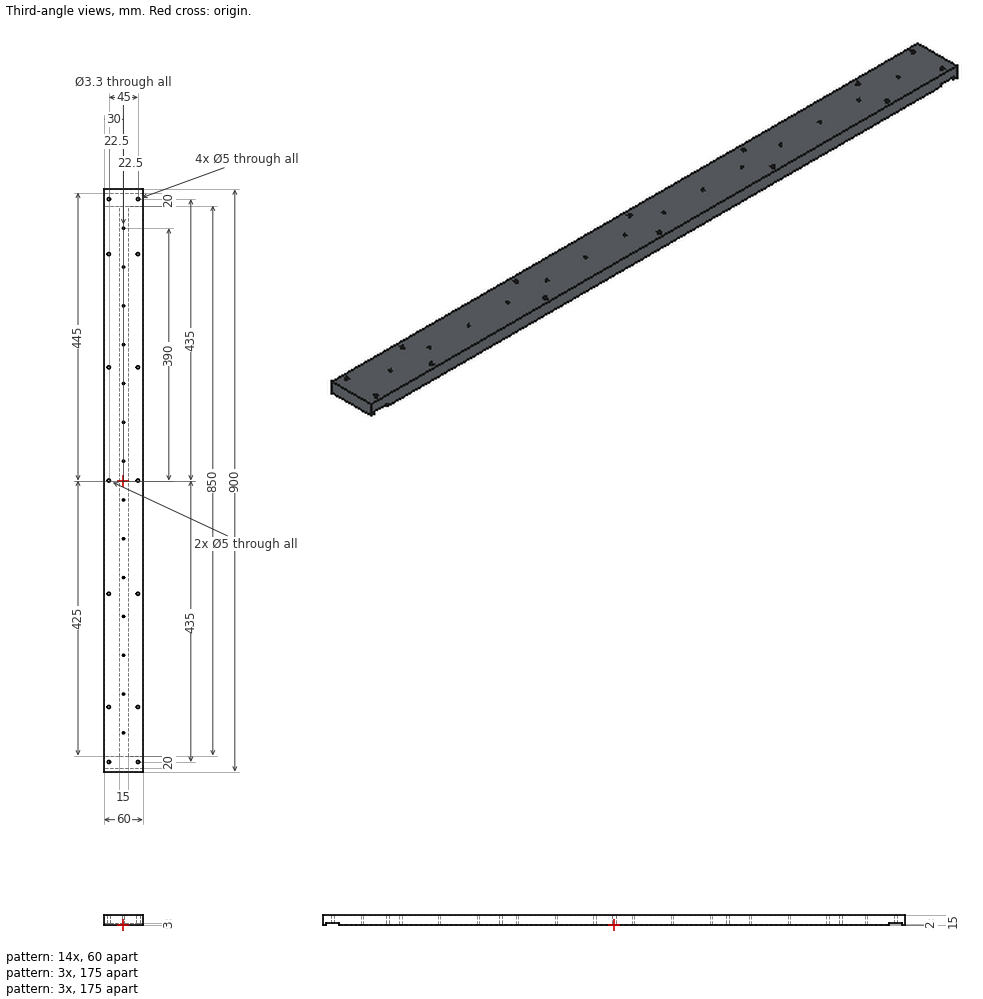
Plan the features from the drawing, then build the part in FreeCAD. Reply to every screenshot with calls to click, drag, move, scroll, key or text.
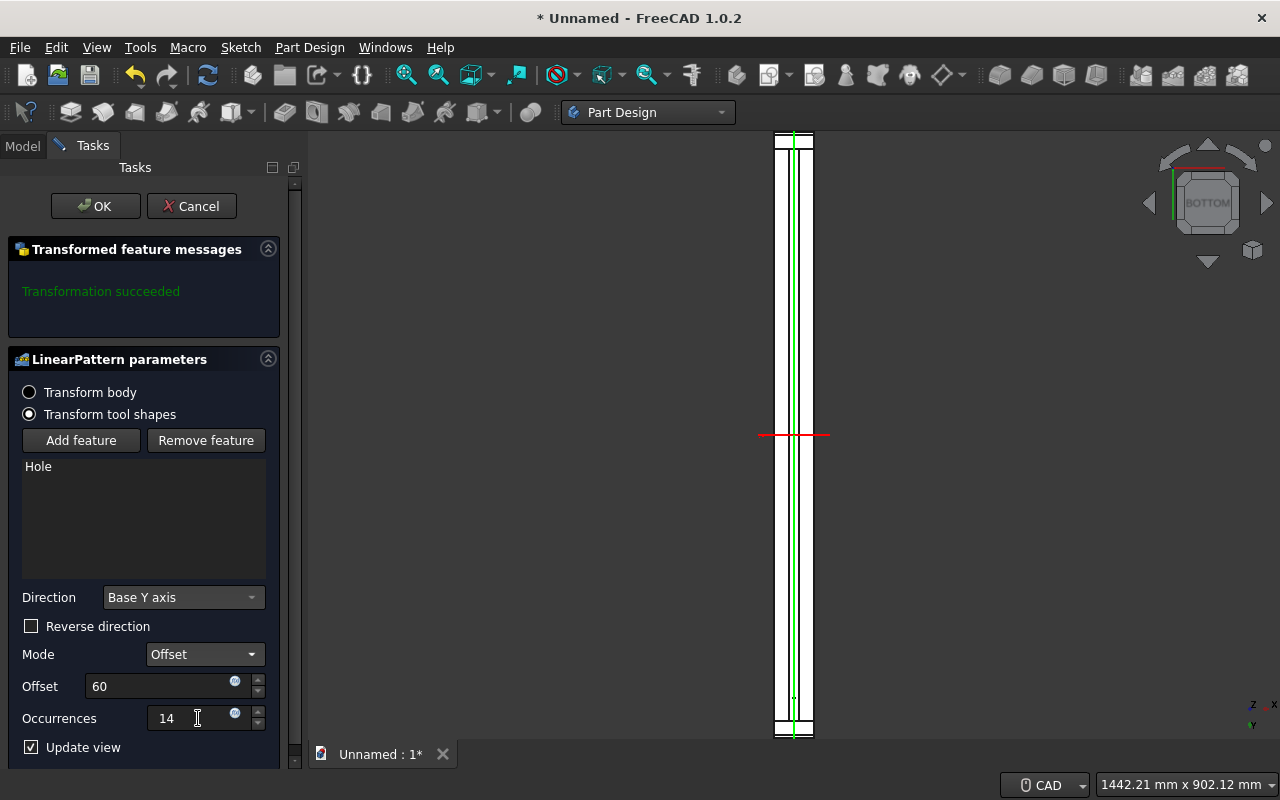
click(30, 626)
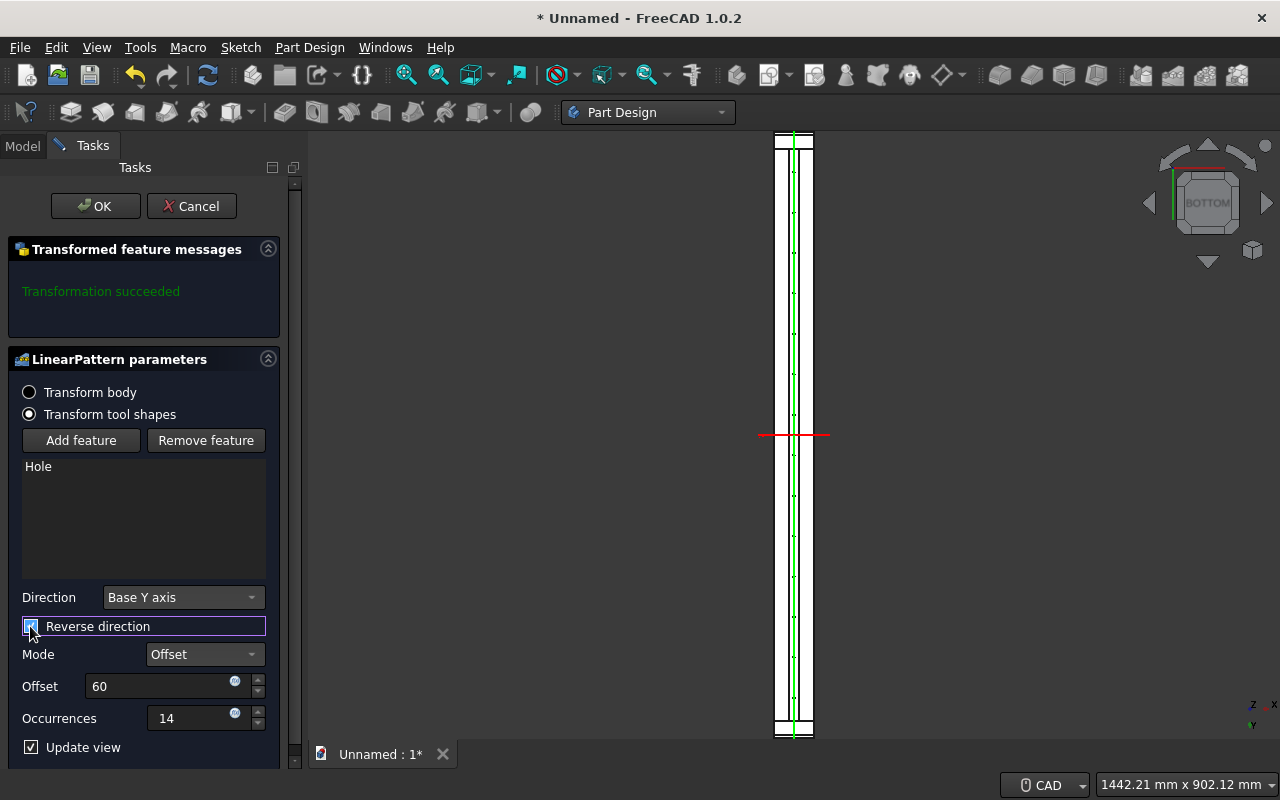
click(96, 206)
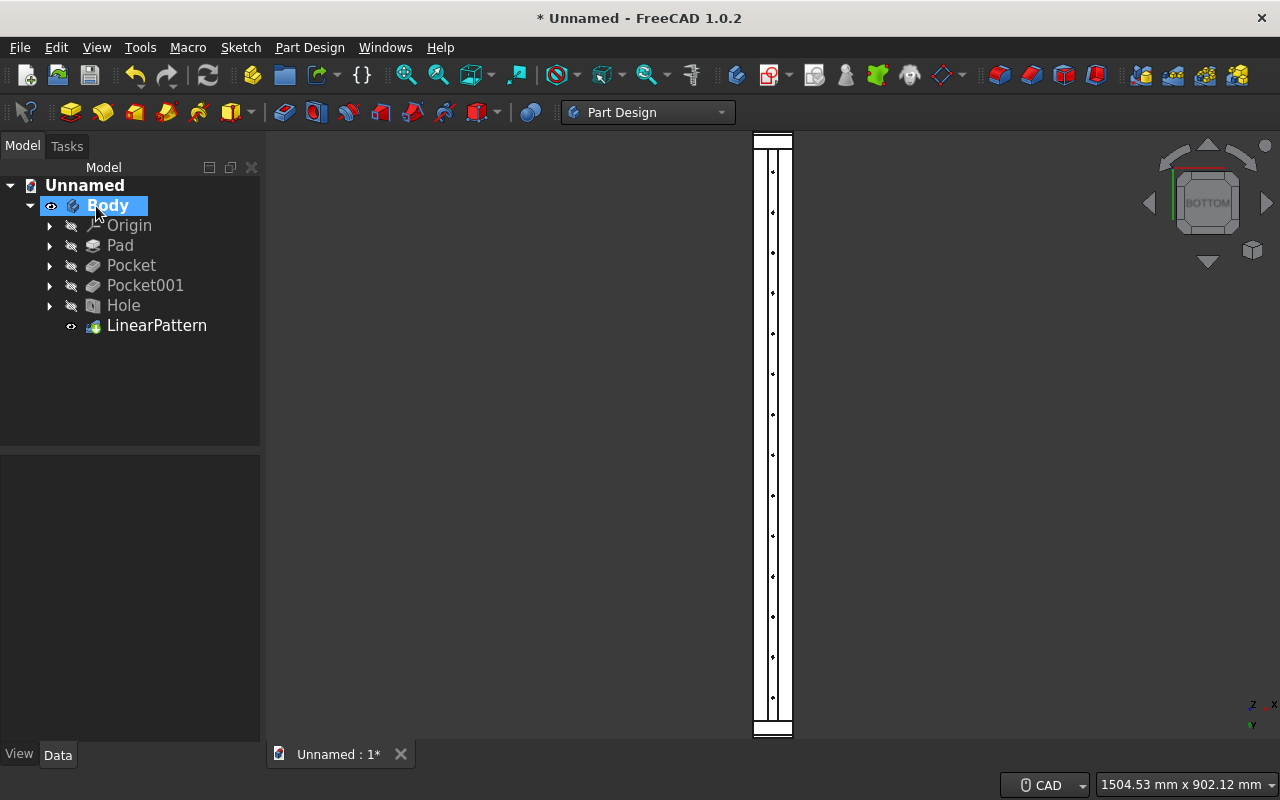
key(1)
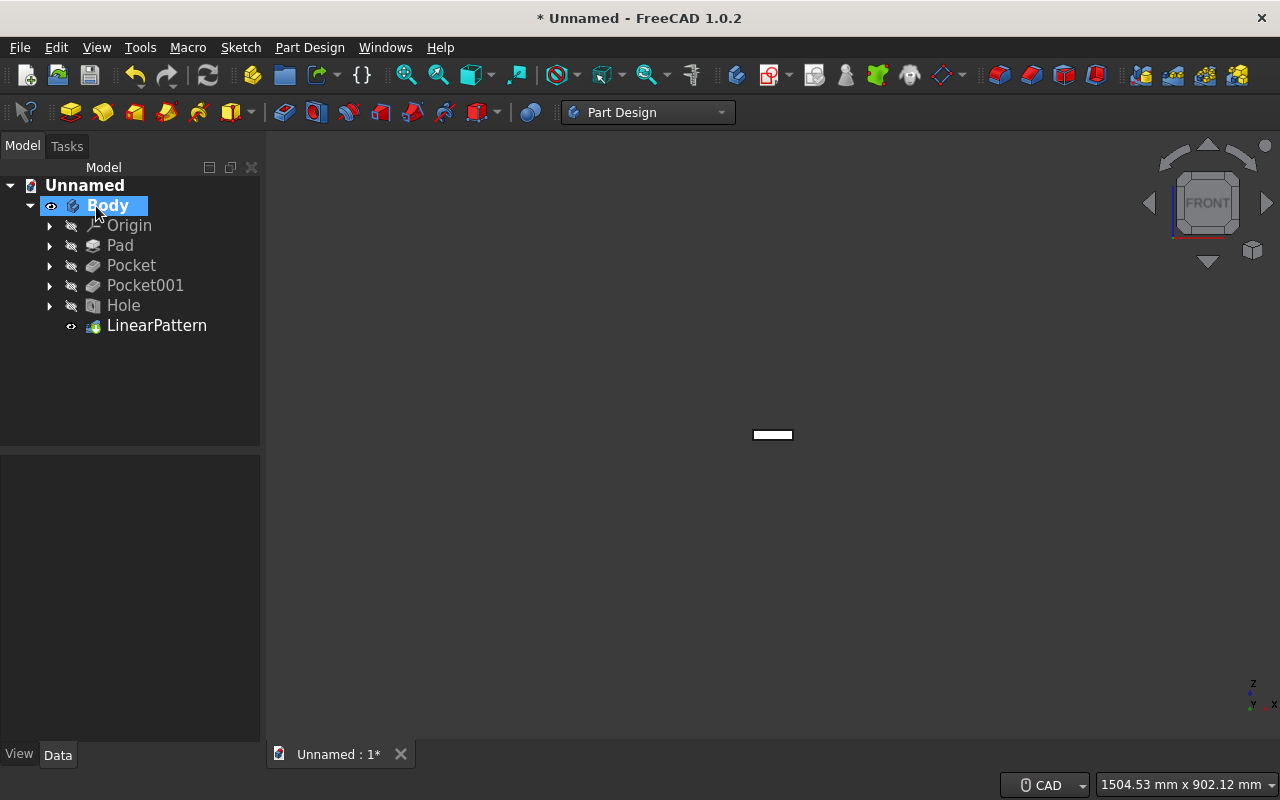
key(v)
key(f)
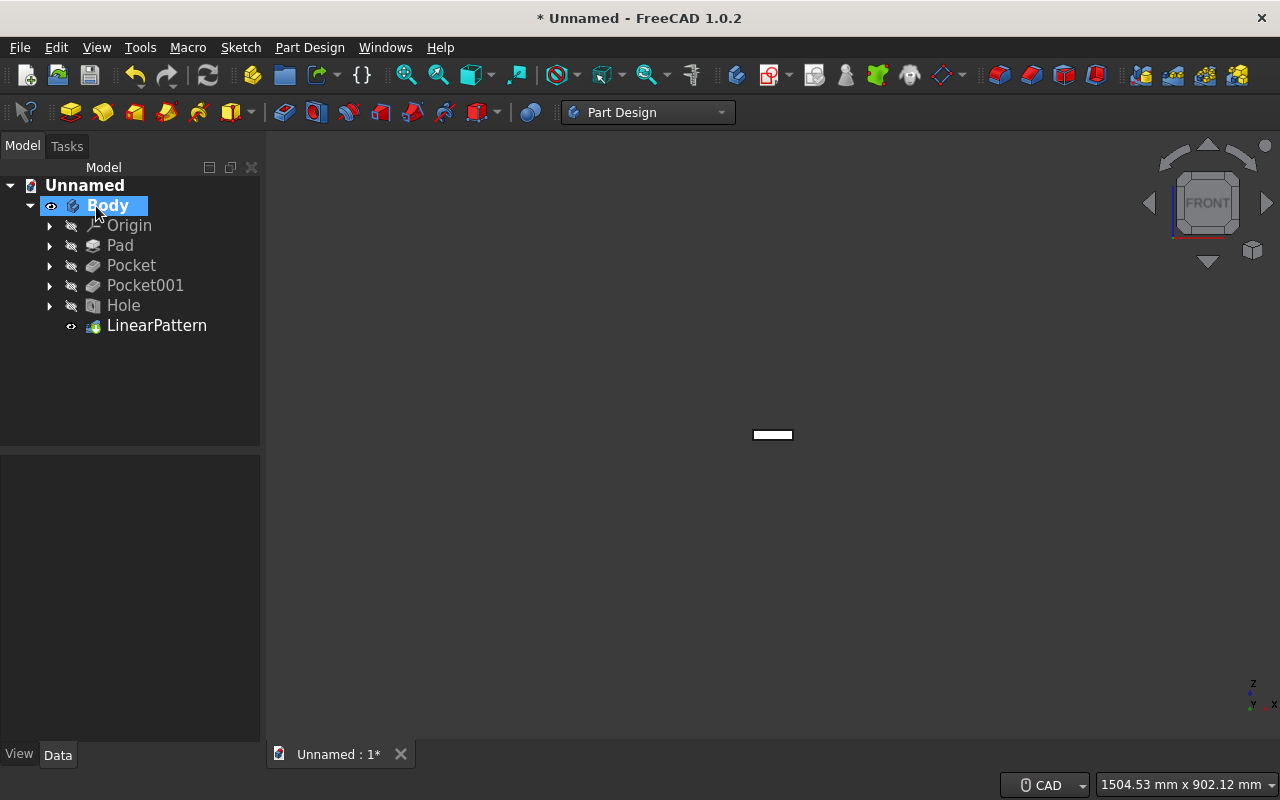
key(5)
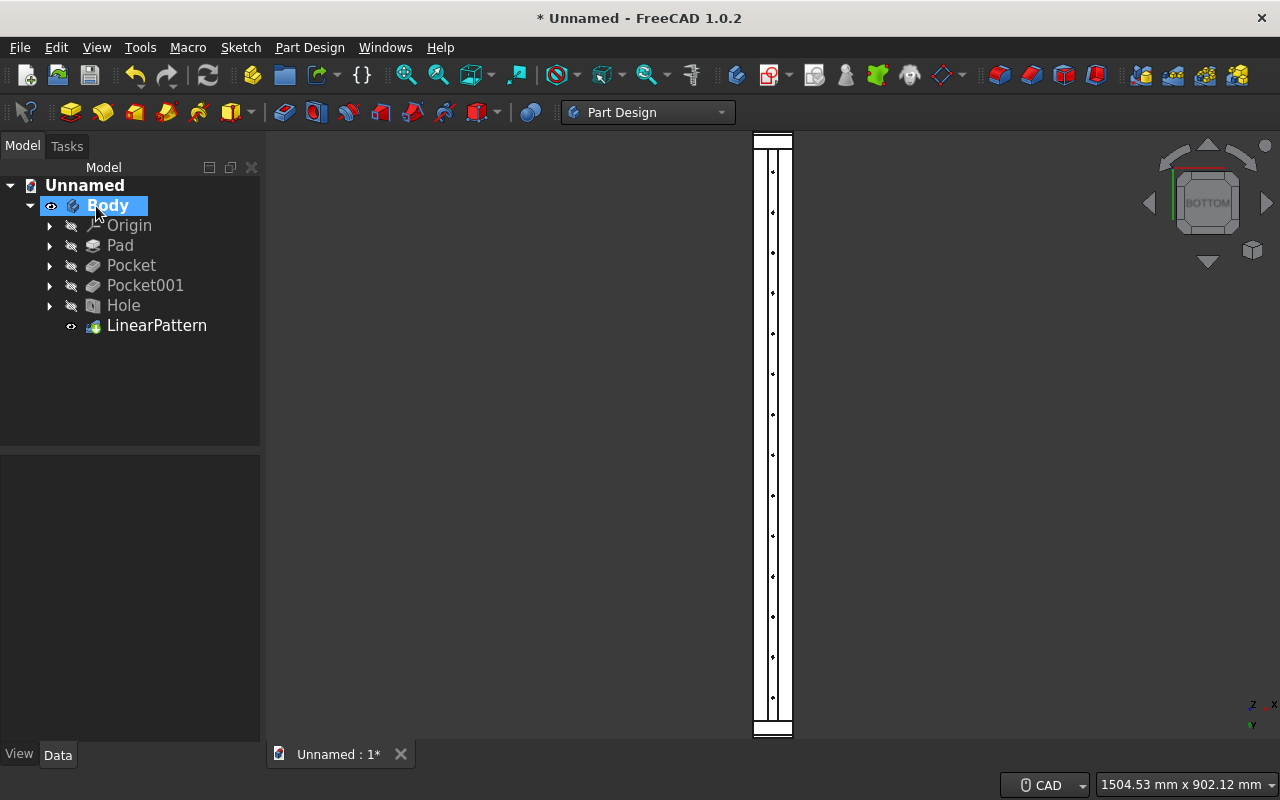
key(3)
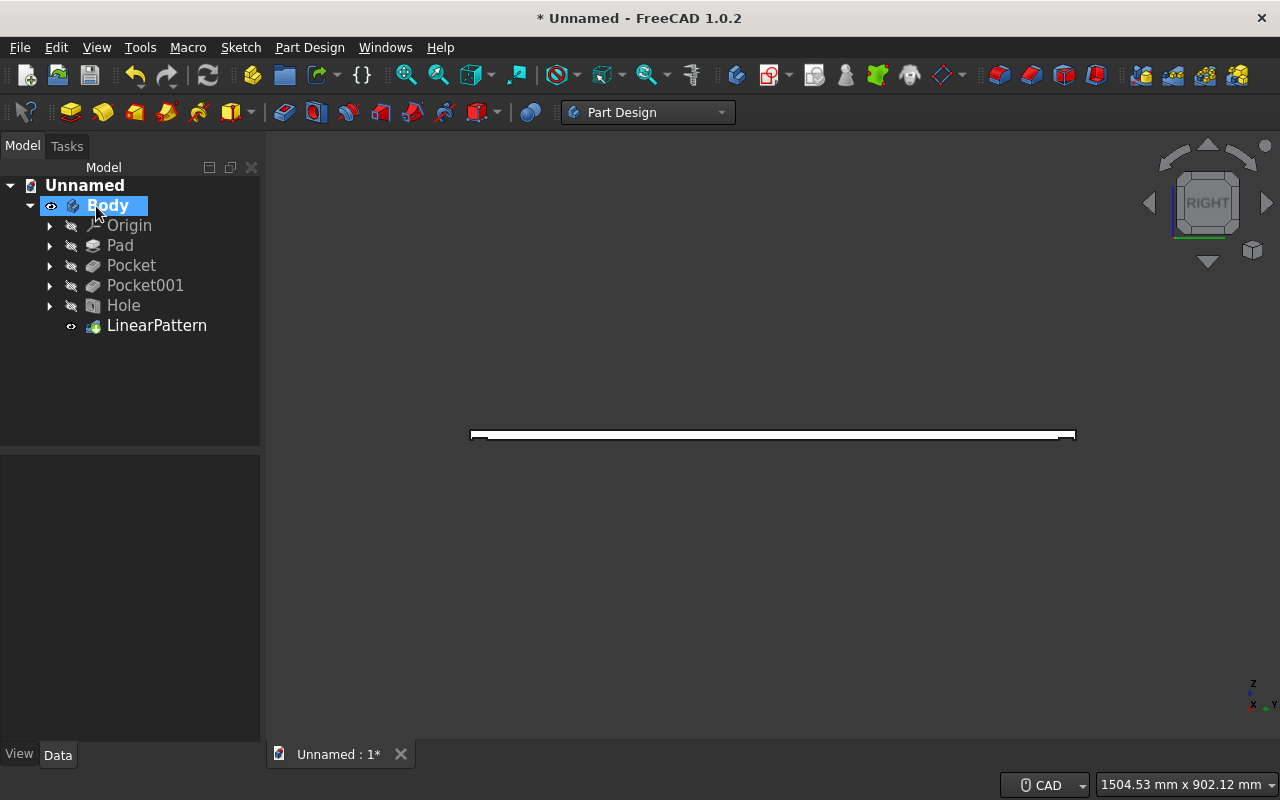
click(50, 226)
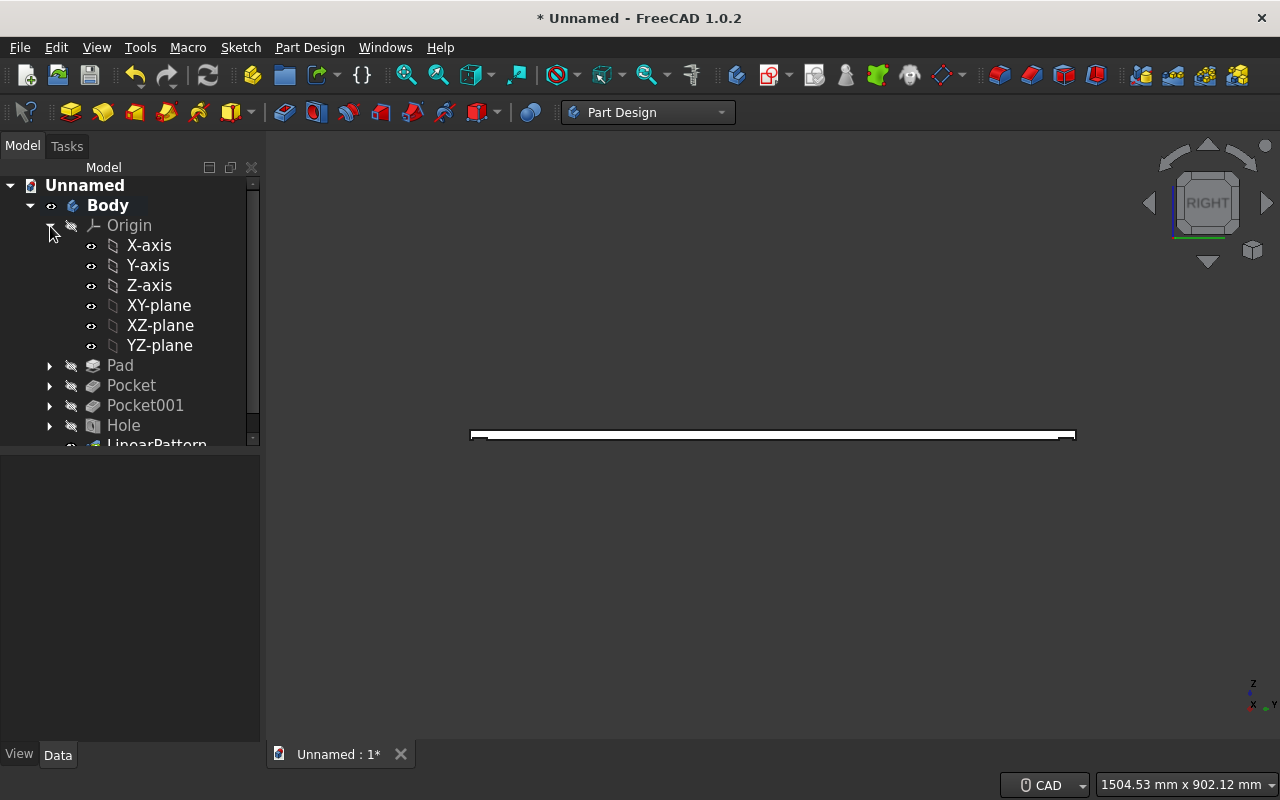
click(136, 306)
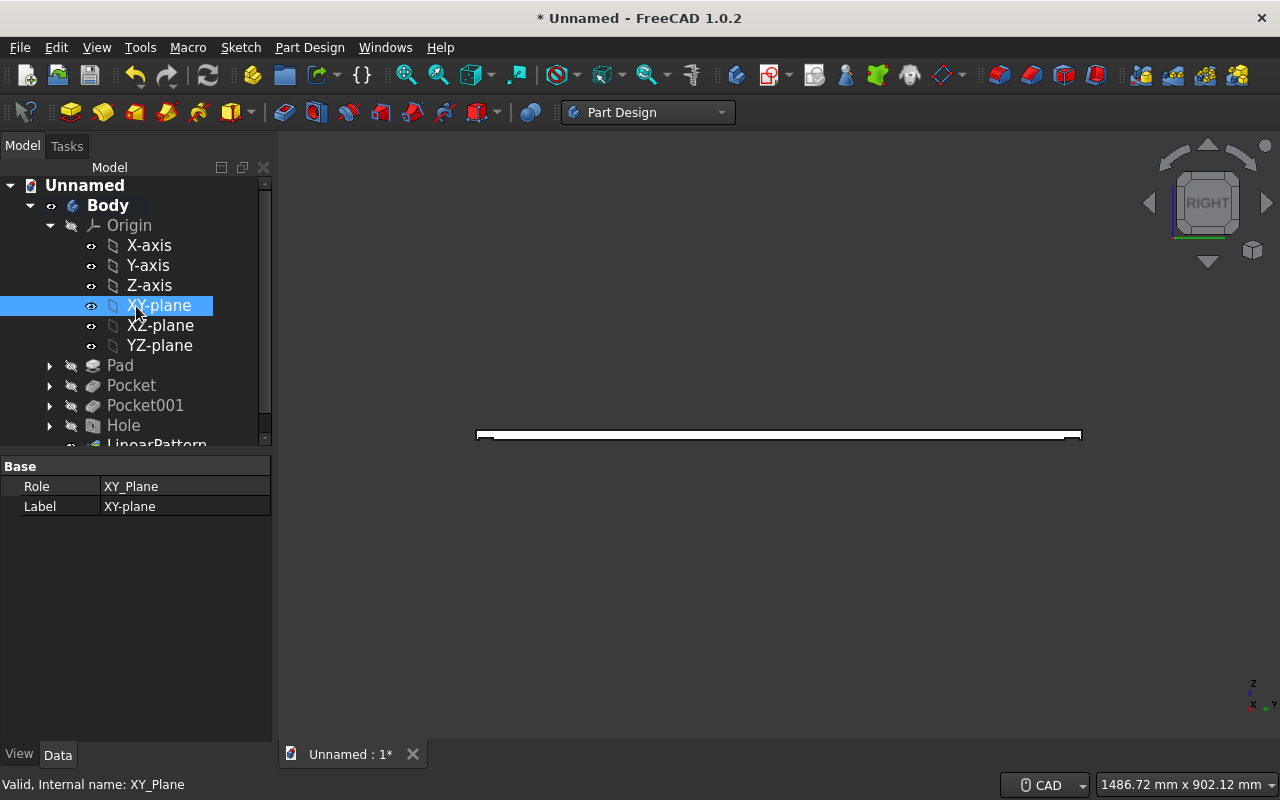
click(942, 76)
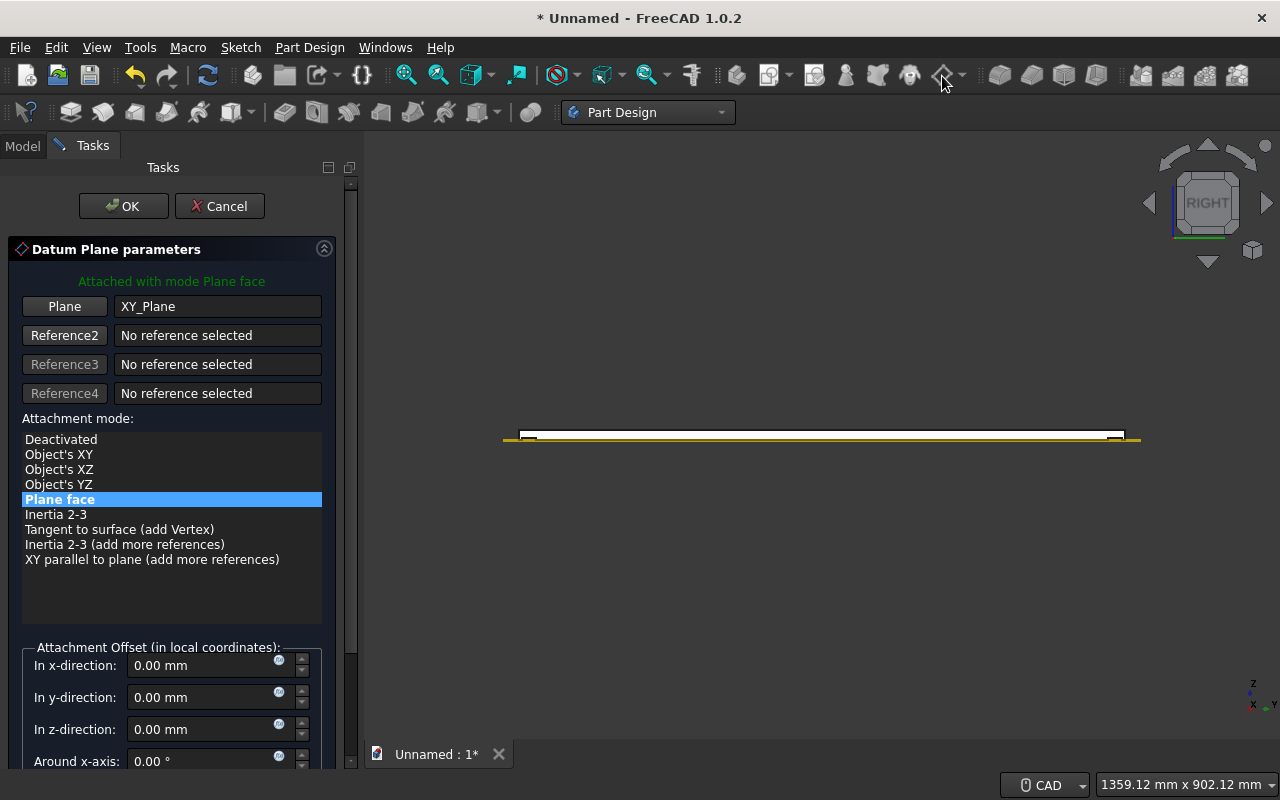
triple_click(210, 729)